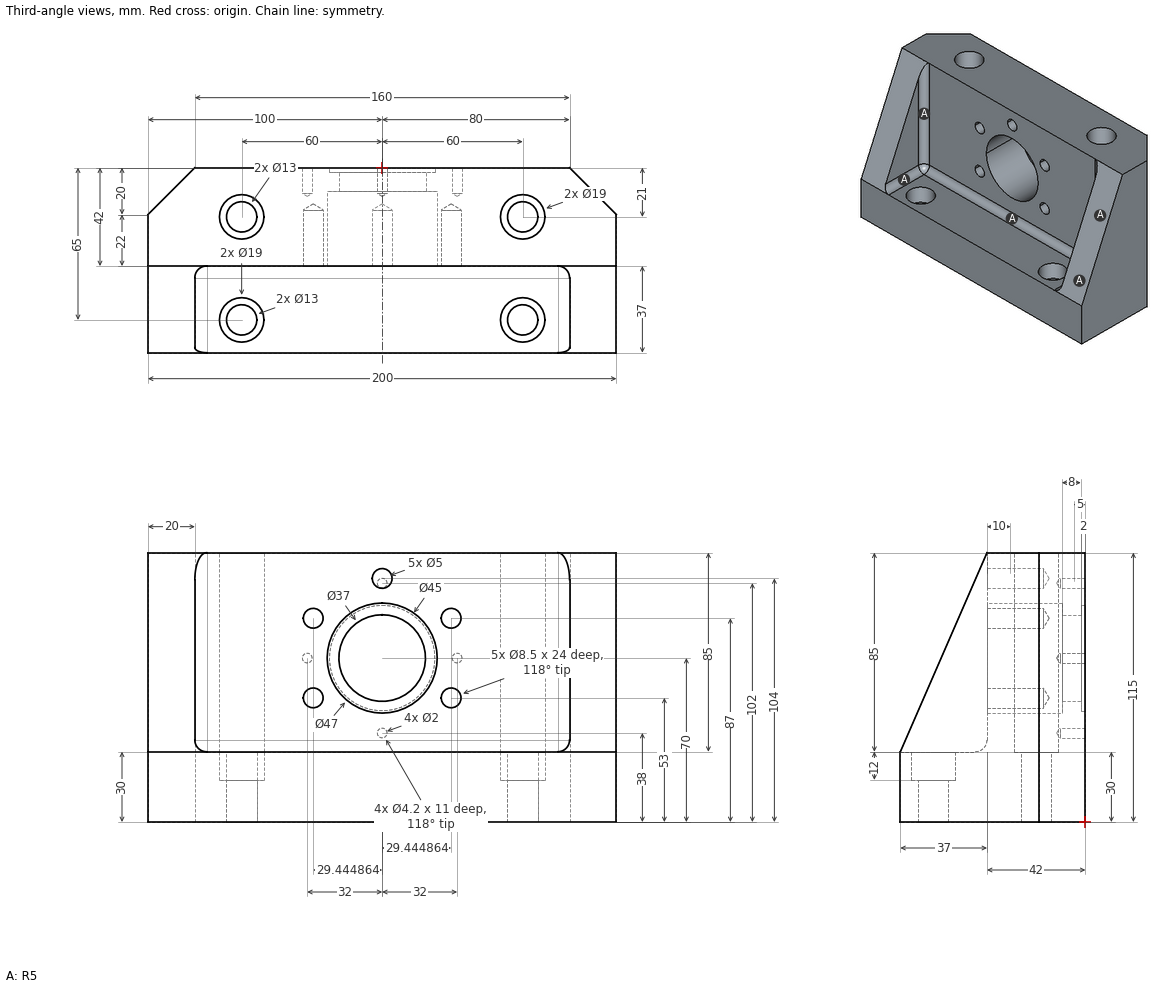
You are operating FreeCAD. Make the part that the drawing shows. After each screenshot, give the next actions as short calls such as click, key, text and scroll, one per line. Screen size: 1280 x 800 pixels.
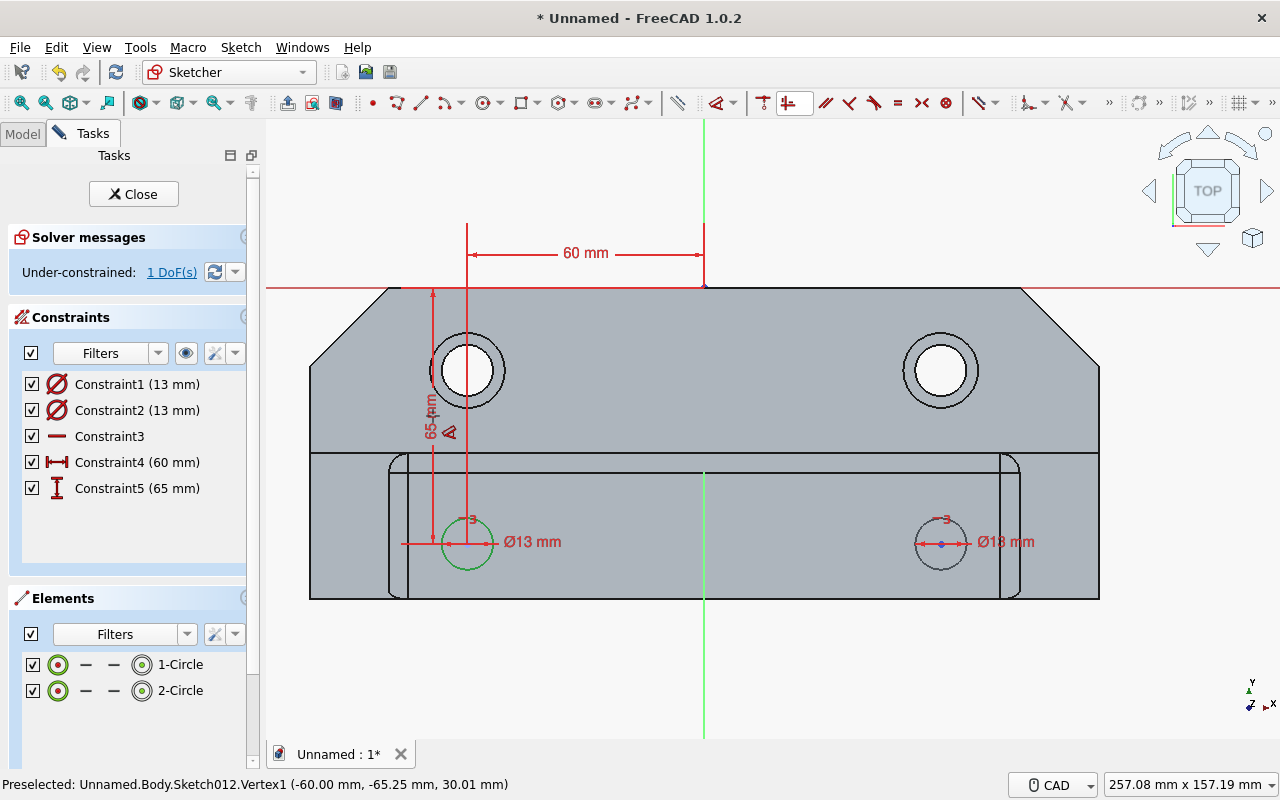
click(941, 544)
click(823, 254)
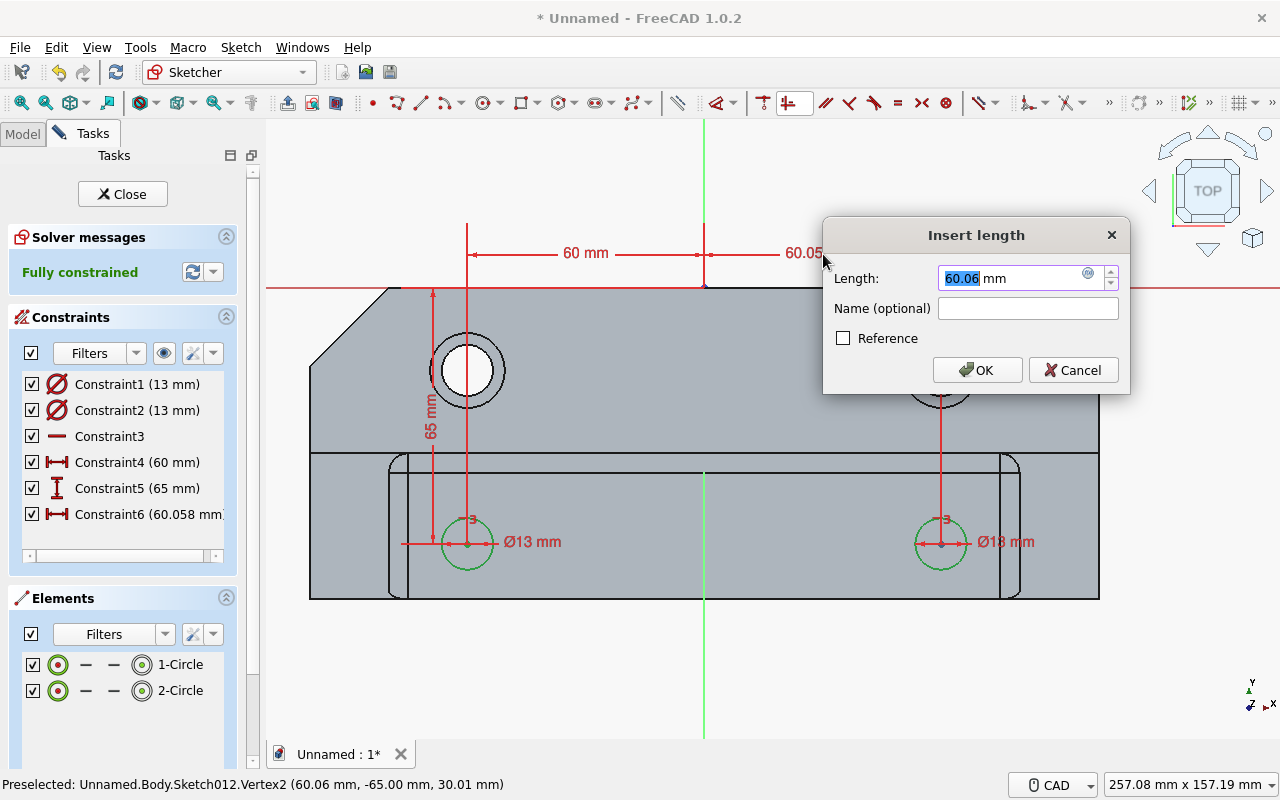
text(60)
key(Return)
key(Escape)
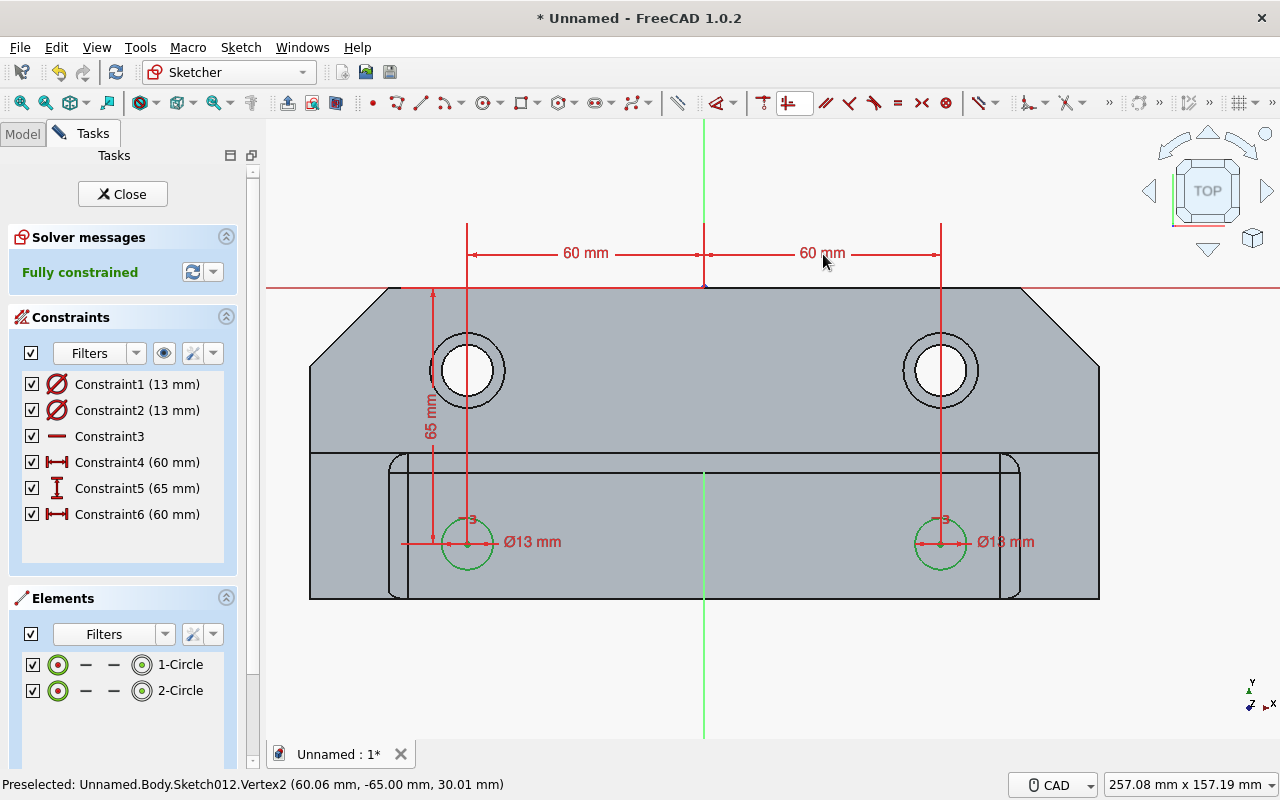
click(123, 194)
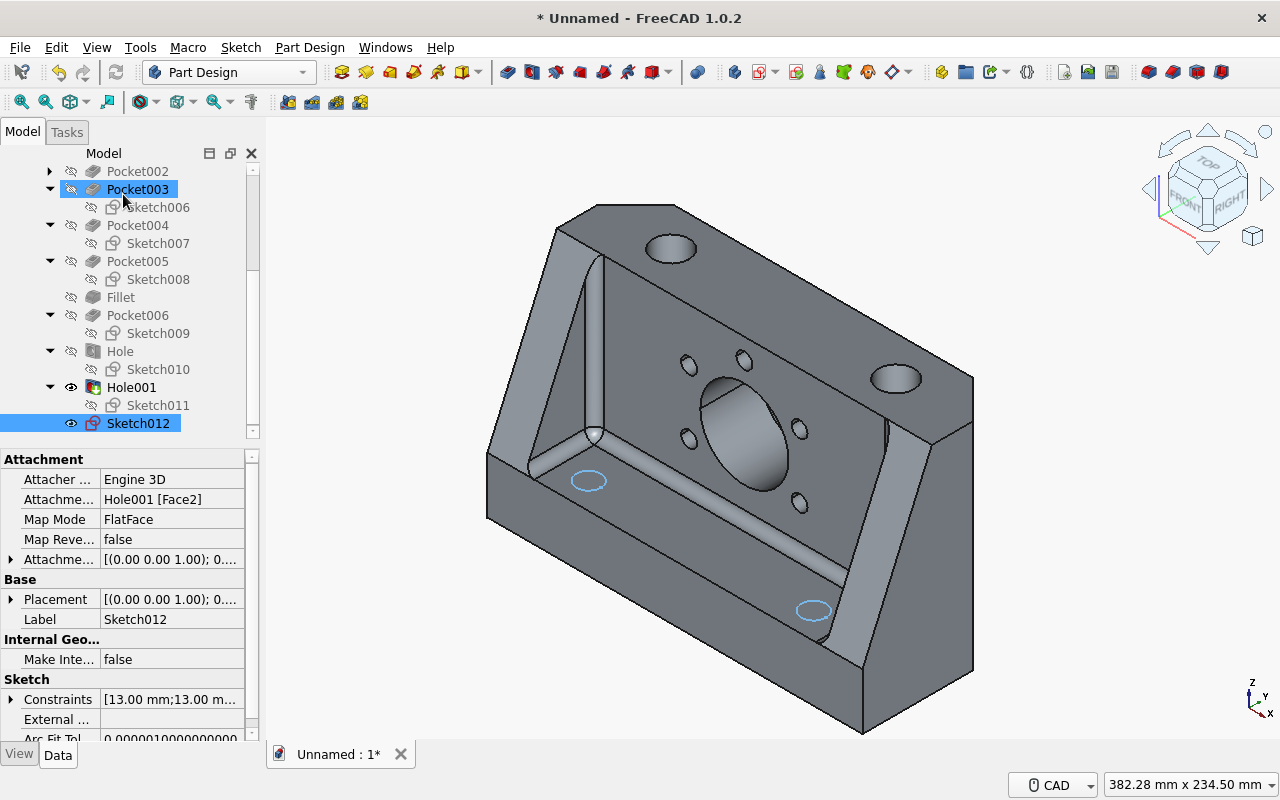
click(508, 72)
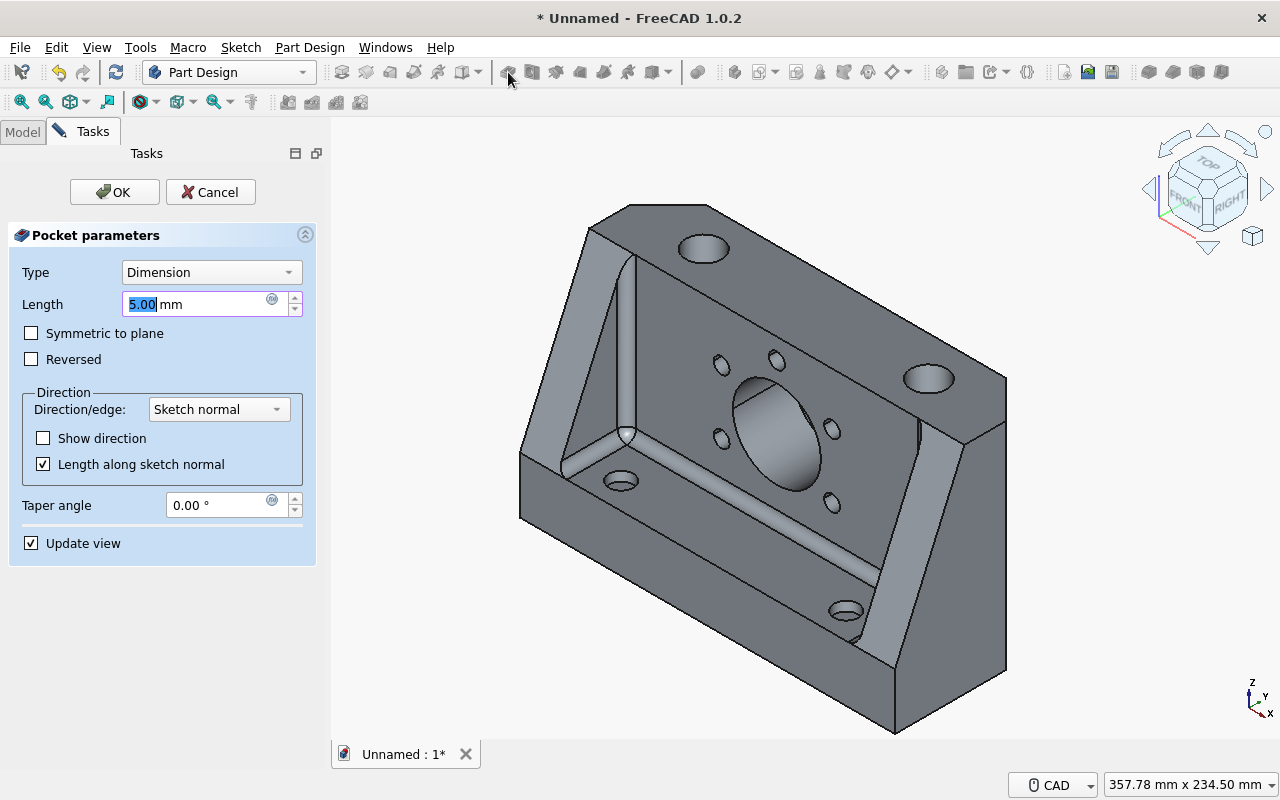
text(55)
key(Tab)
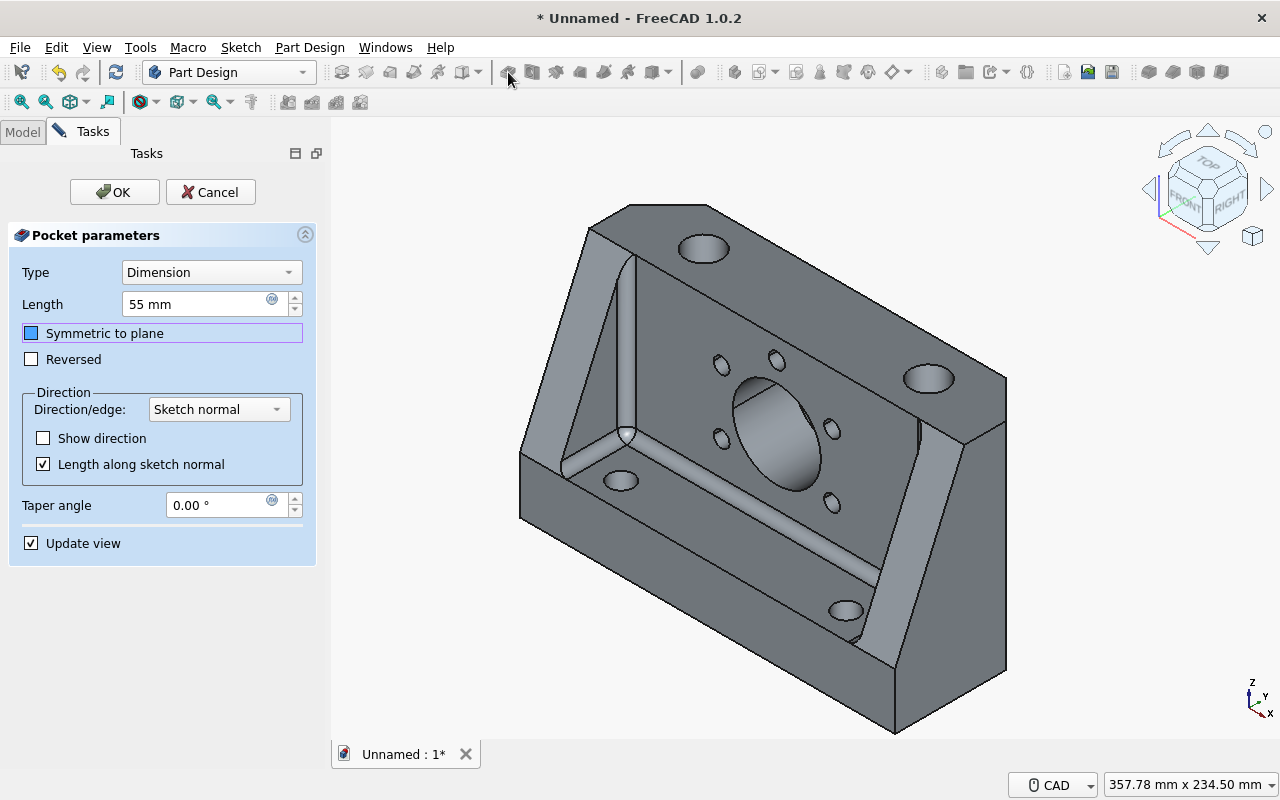
click(115, 192)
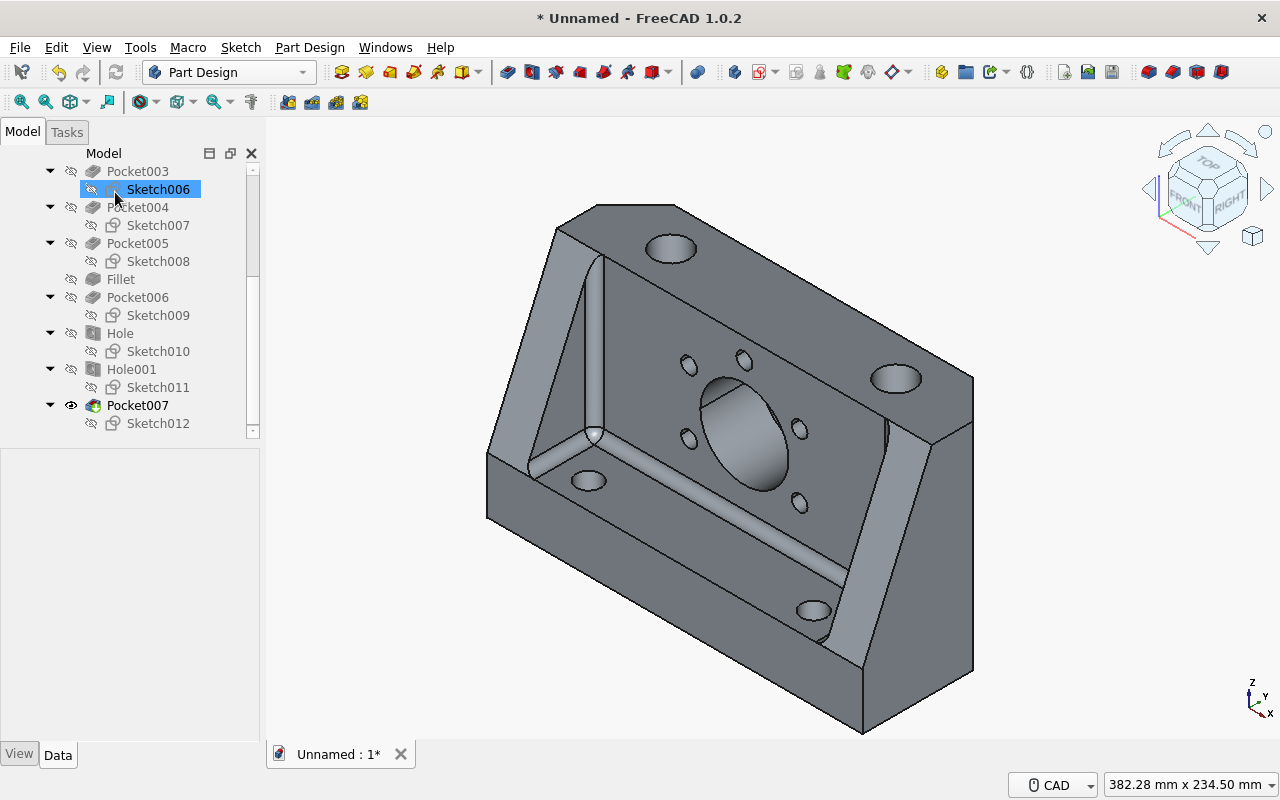
click(745, 566)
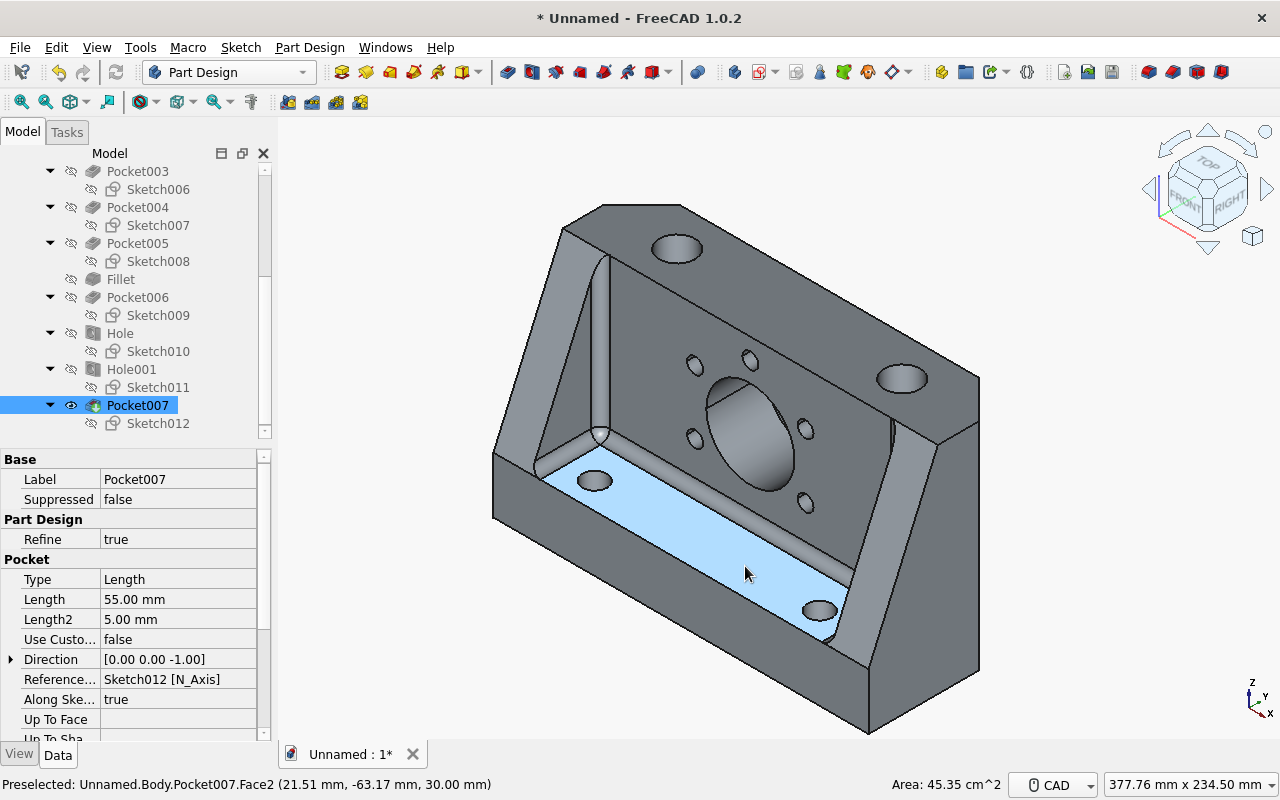
click(760, 72)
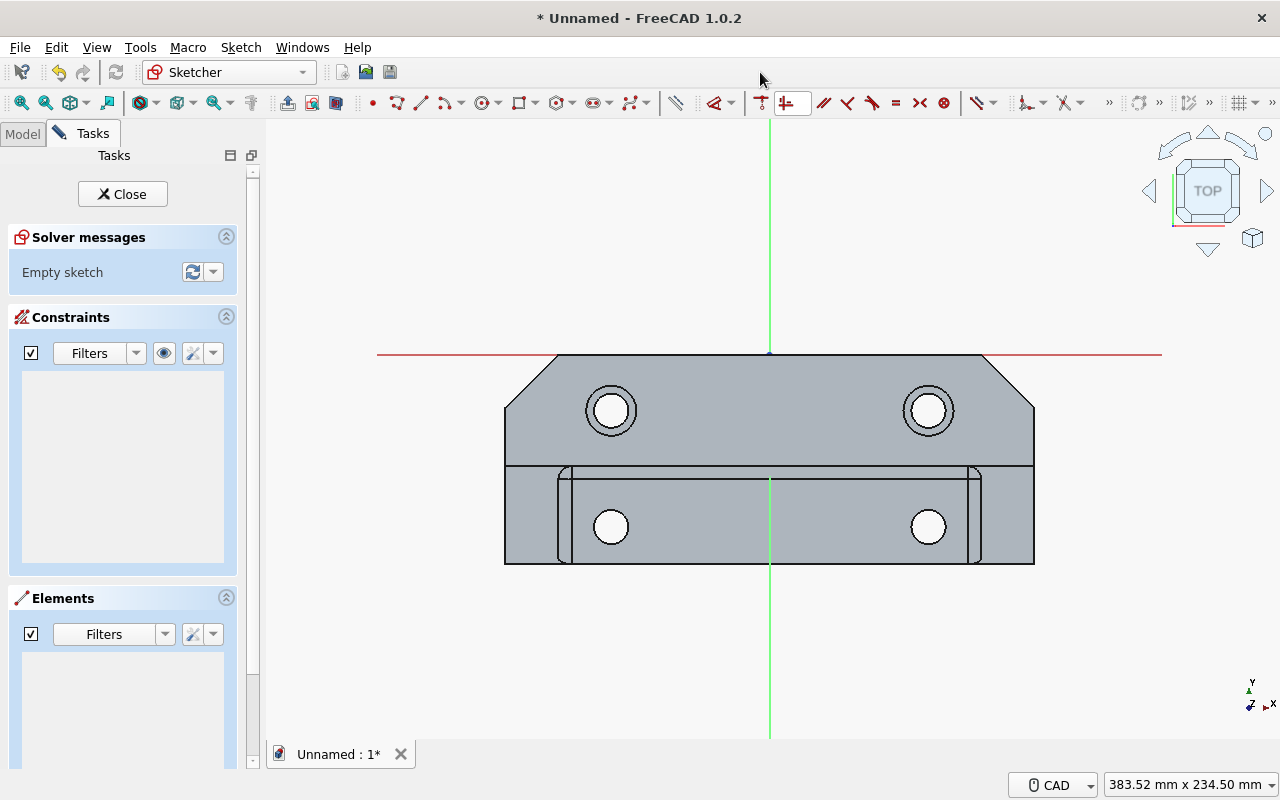
scroll(903, 504, up, 2)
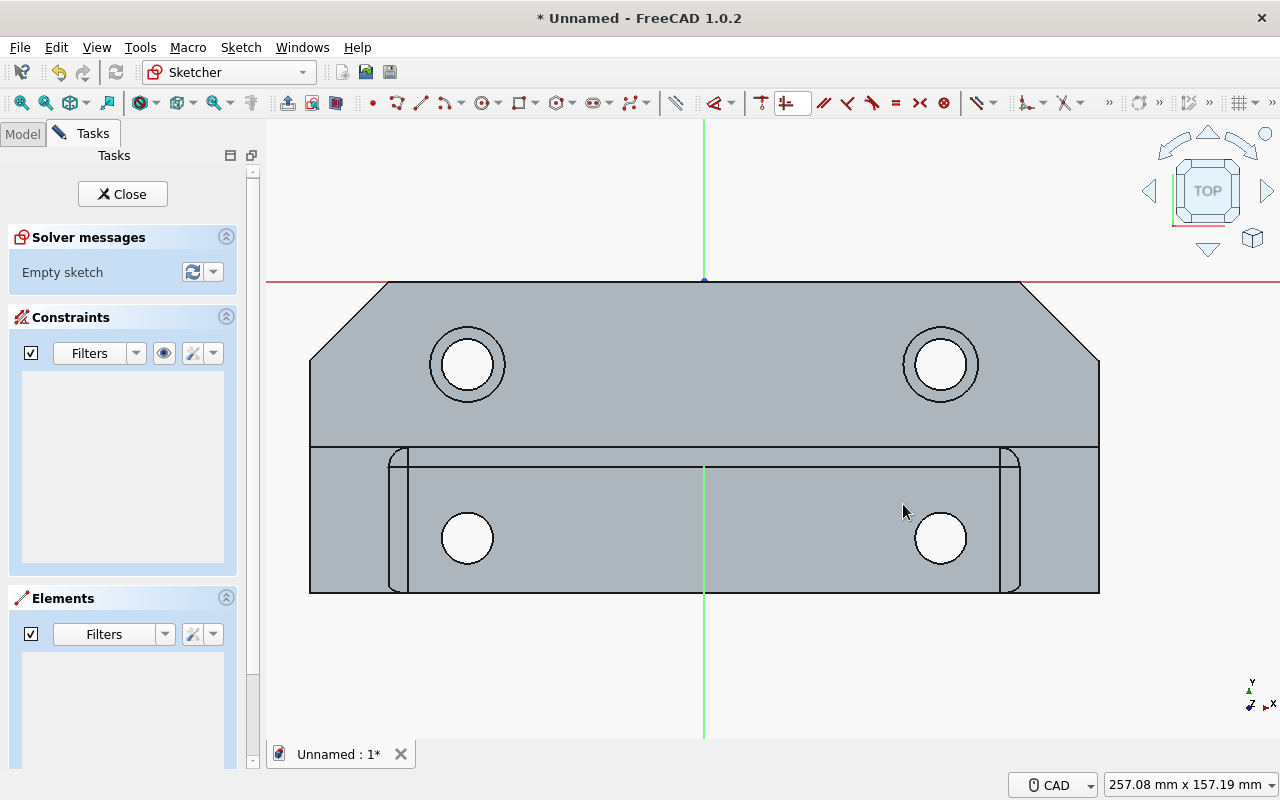
key(g)
key(c)